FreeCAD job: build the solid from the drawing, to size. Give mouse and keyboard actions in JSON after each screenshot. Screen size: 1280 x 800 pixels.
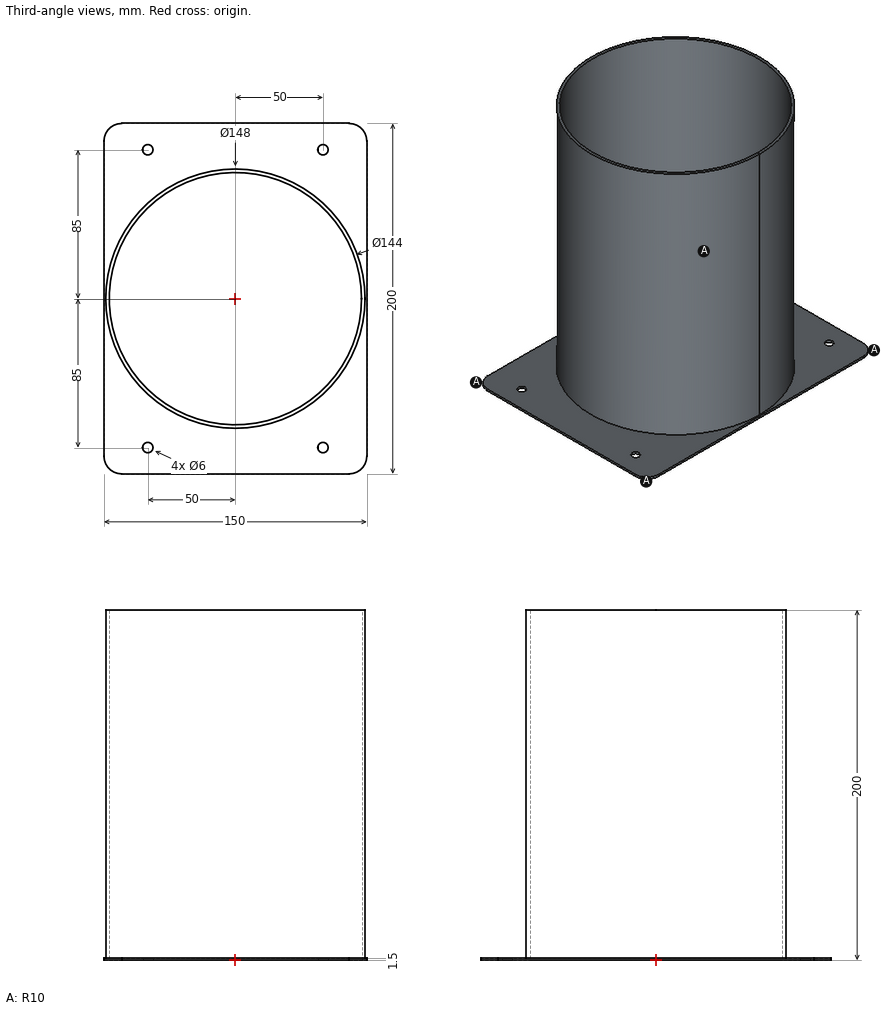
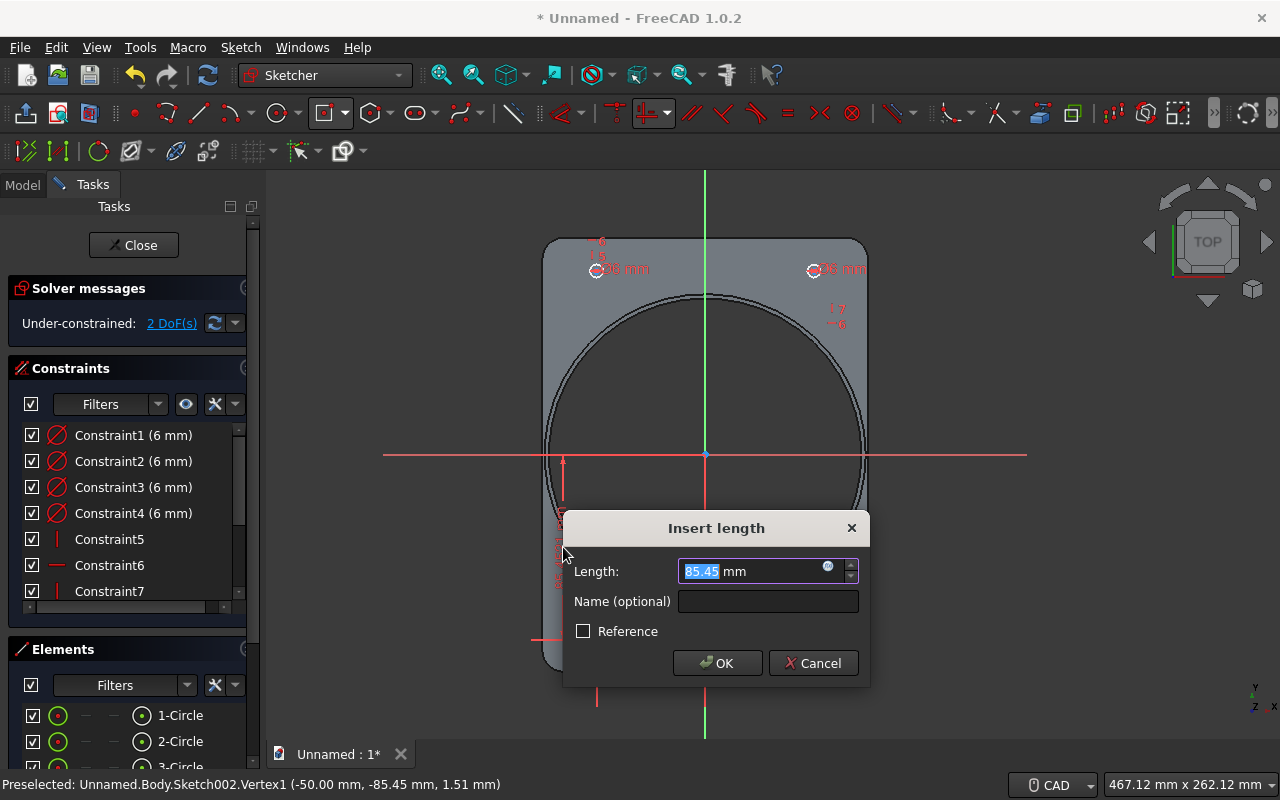
{"action": "type", "text": "85"}
{"action": "key", "text": "Return"}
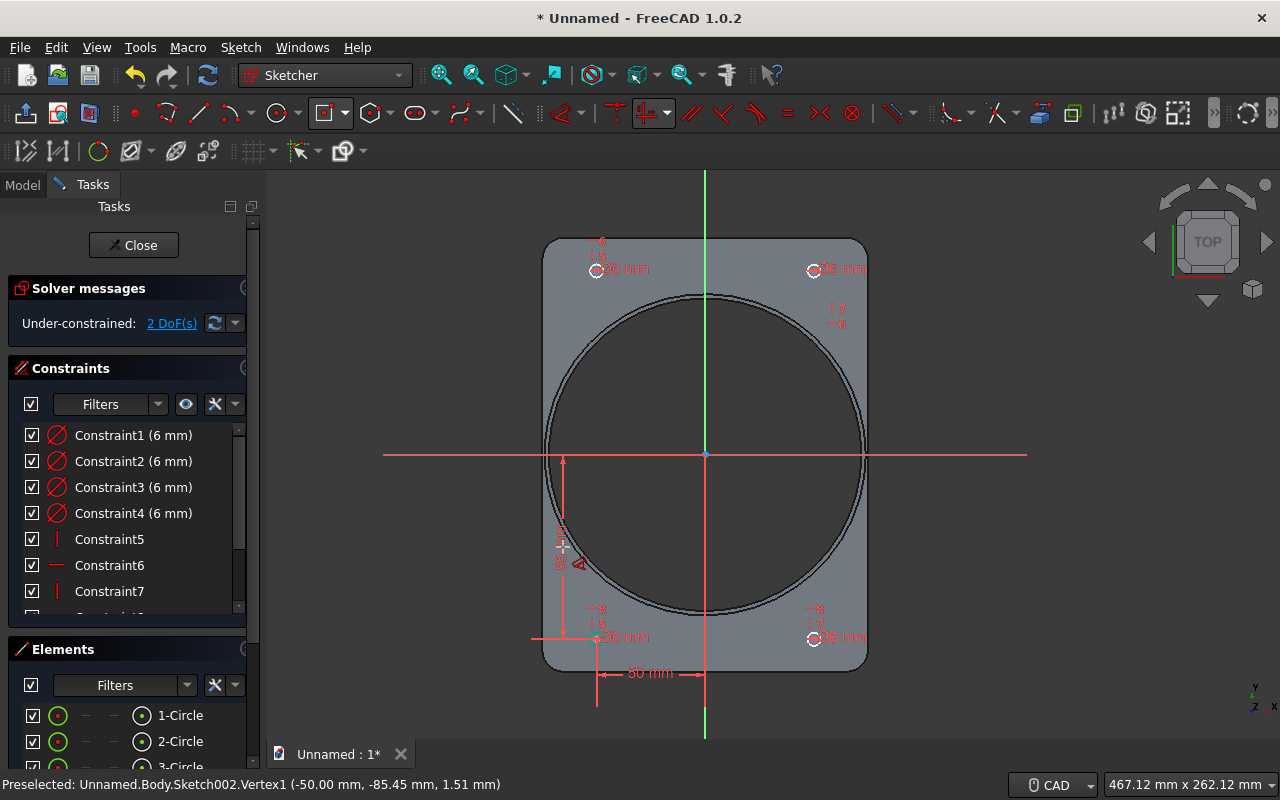
{"action": "left_click", "coordinate": [597, 271]}
{"action": "left_click", "coordinate": [563, 363]}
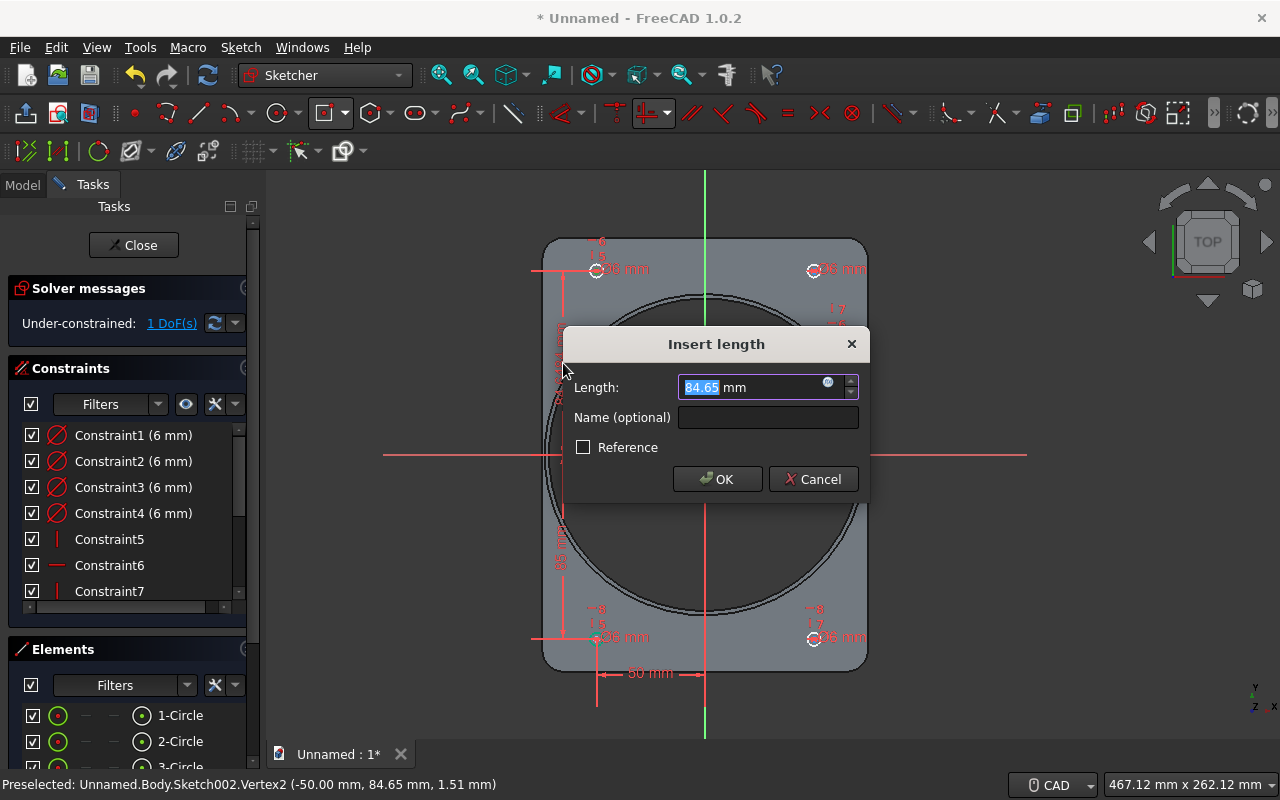
{"action": "type", "text": "85"}
{"action": "key", "text": "Return"}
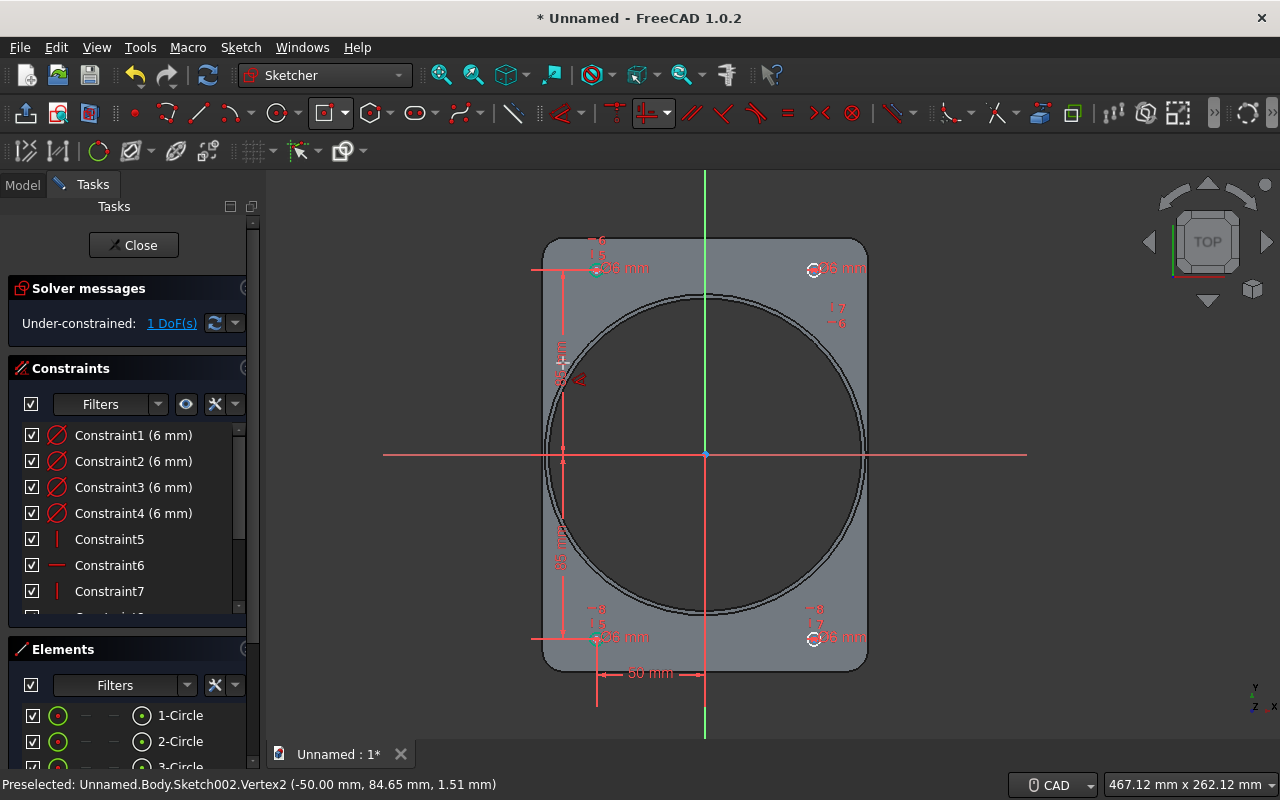
{"action": "left_click", "coordinate": [814, 270]}
{"action": "left_click", "coordinate": [760, 236]}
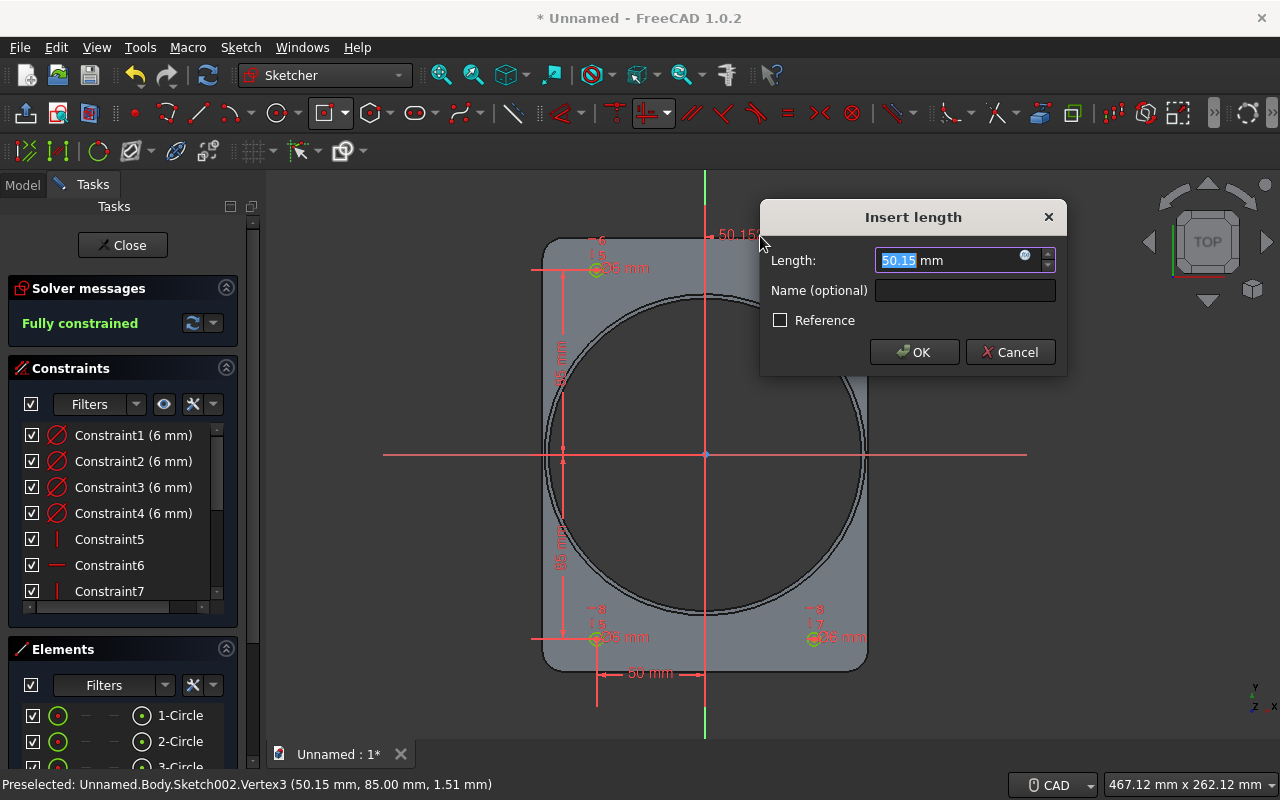
{"action": "type", "text": "50"}
{"action": "key", "text": "Return"}
{"action": "key", "text": "Escape"}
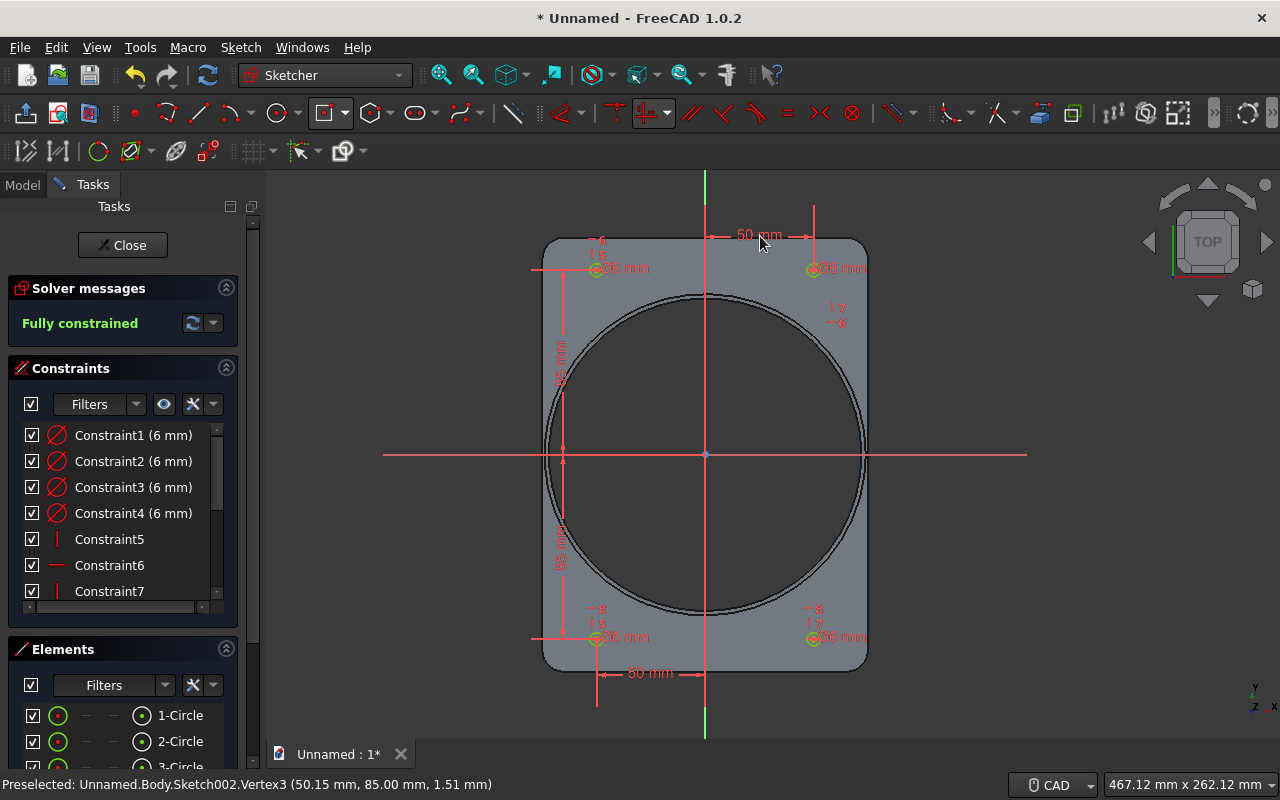
{"action": "left_click", "coordinate": [123, 245]}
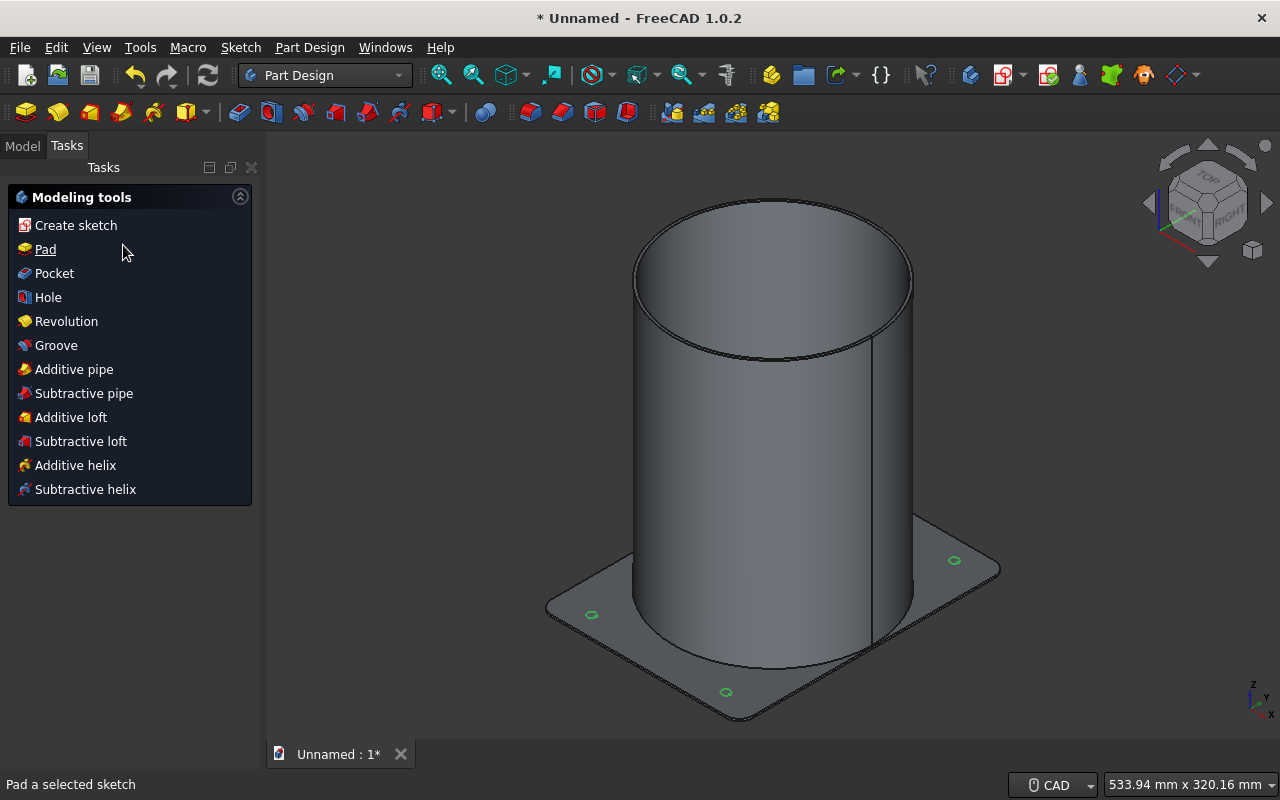
{"action": "left_click", "coordinate": [240, 112]}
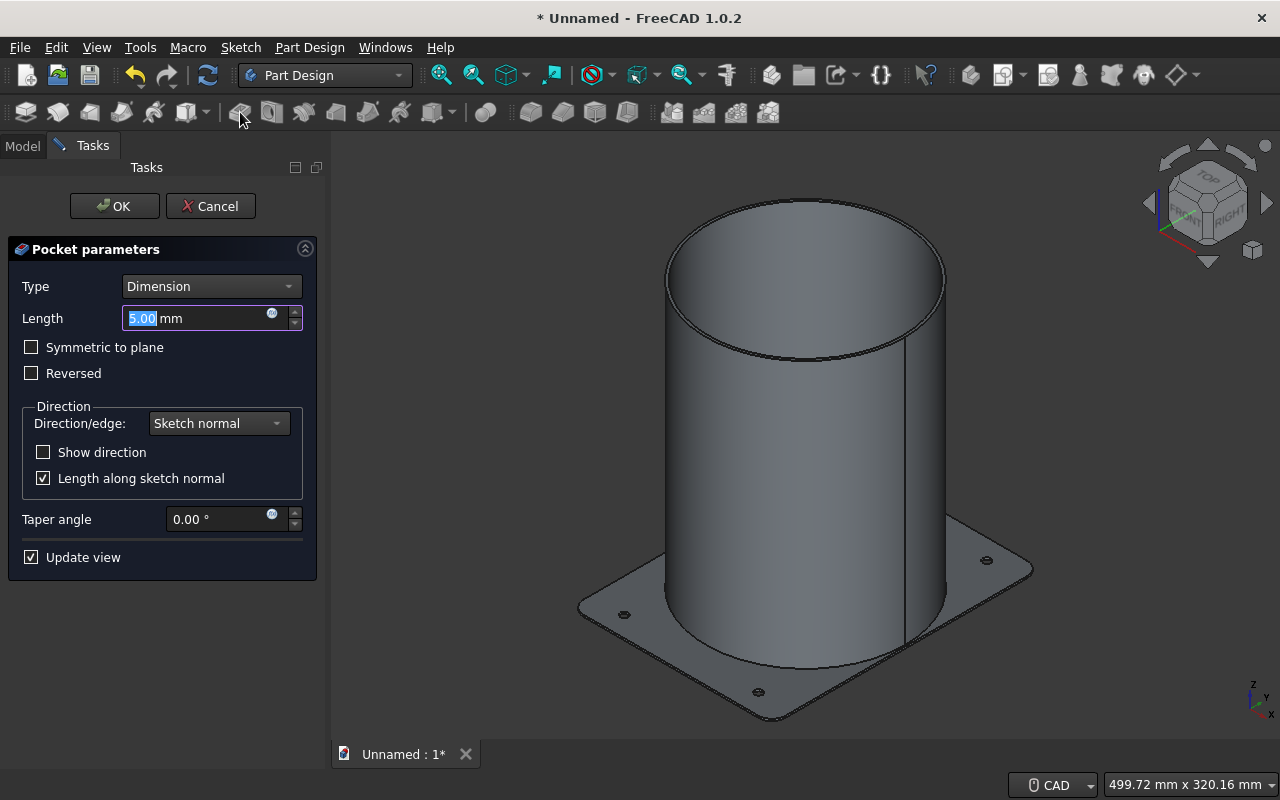
{"action": "left_click", "coordinate": [212, 286]}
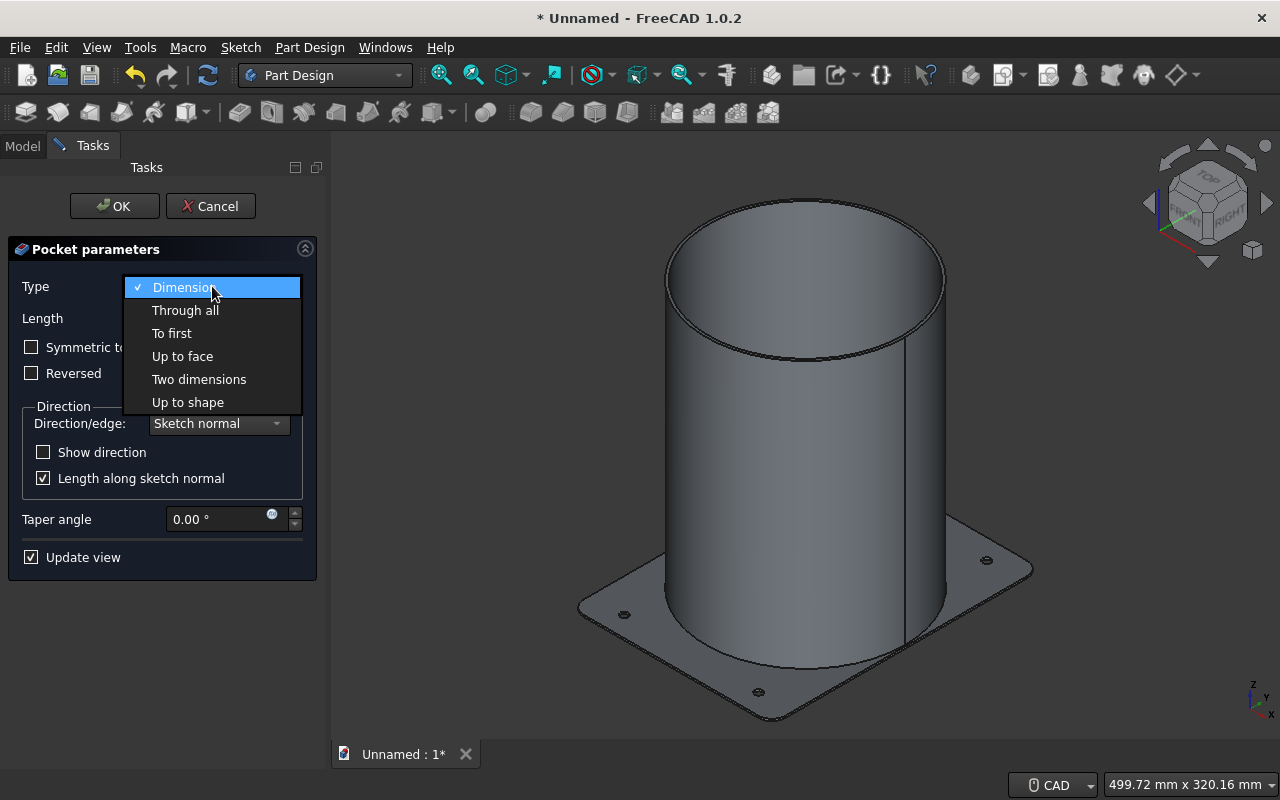
{"action": "left_click", "coordinate": [212, 310]}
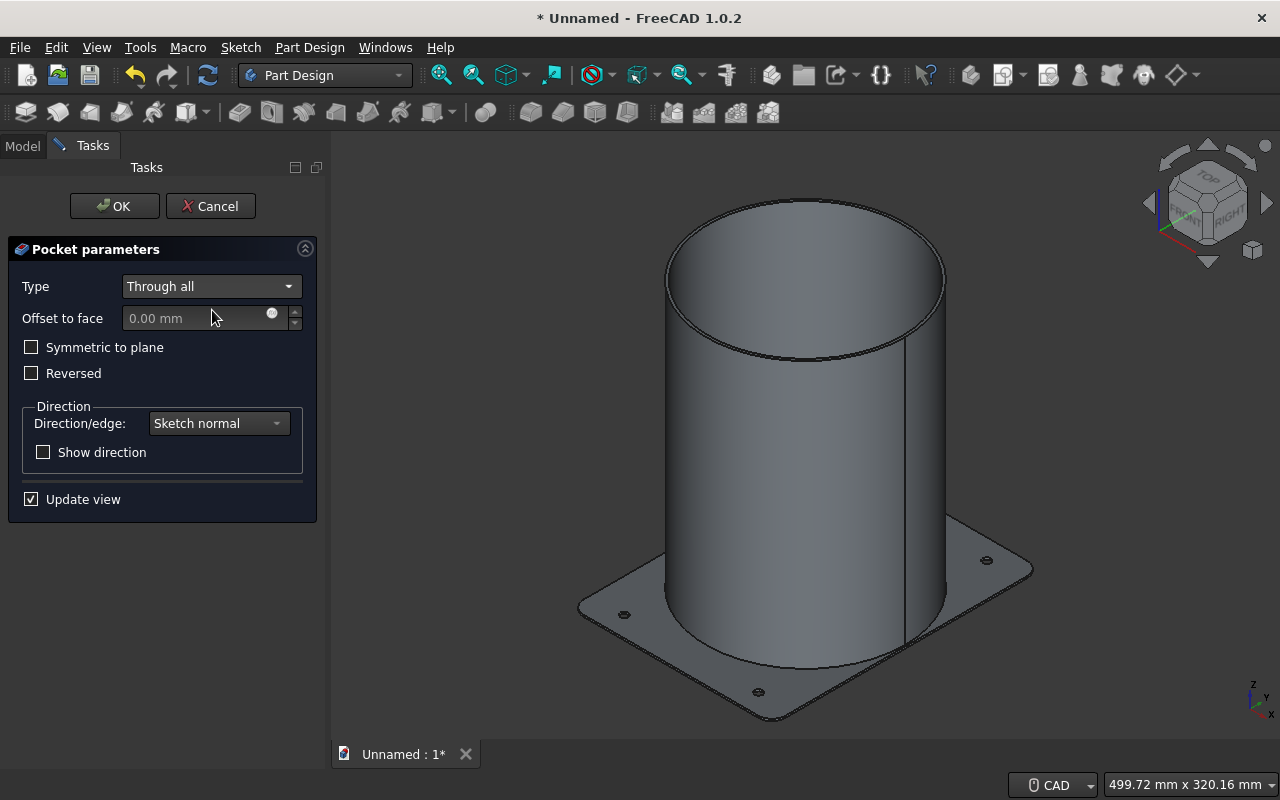
{"action": "left_click", "coordinate": [115, 206]}